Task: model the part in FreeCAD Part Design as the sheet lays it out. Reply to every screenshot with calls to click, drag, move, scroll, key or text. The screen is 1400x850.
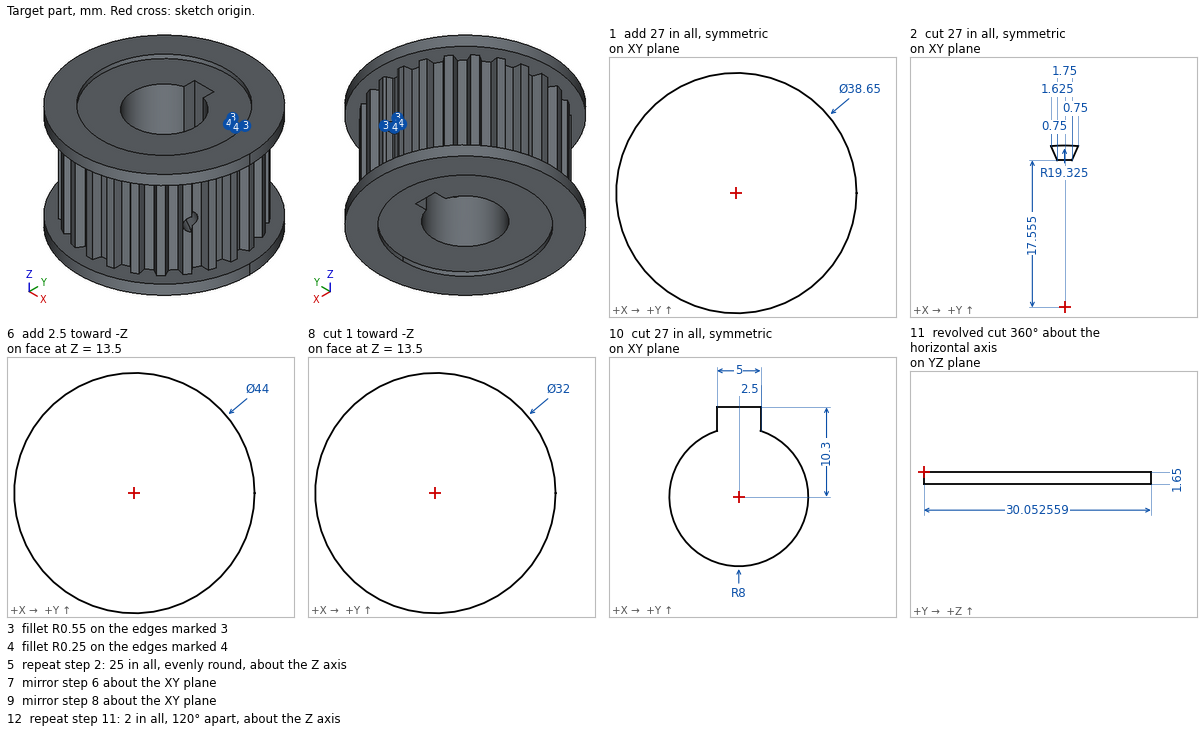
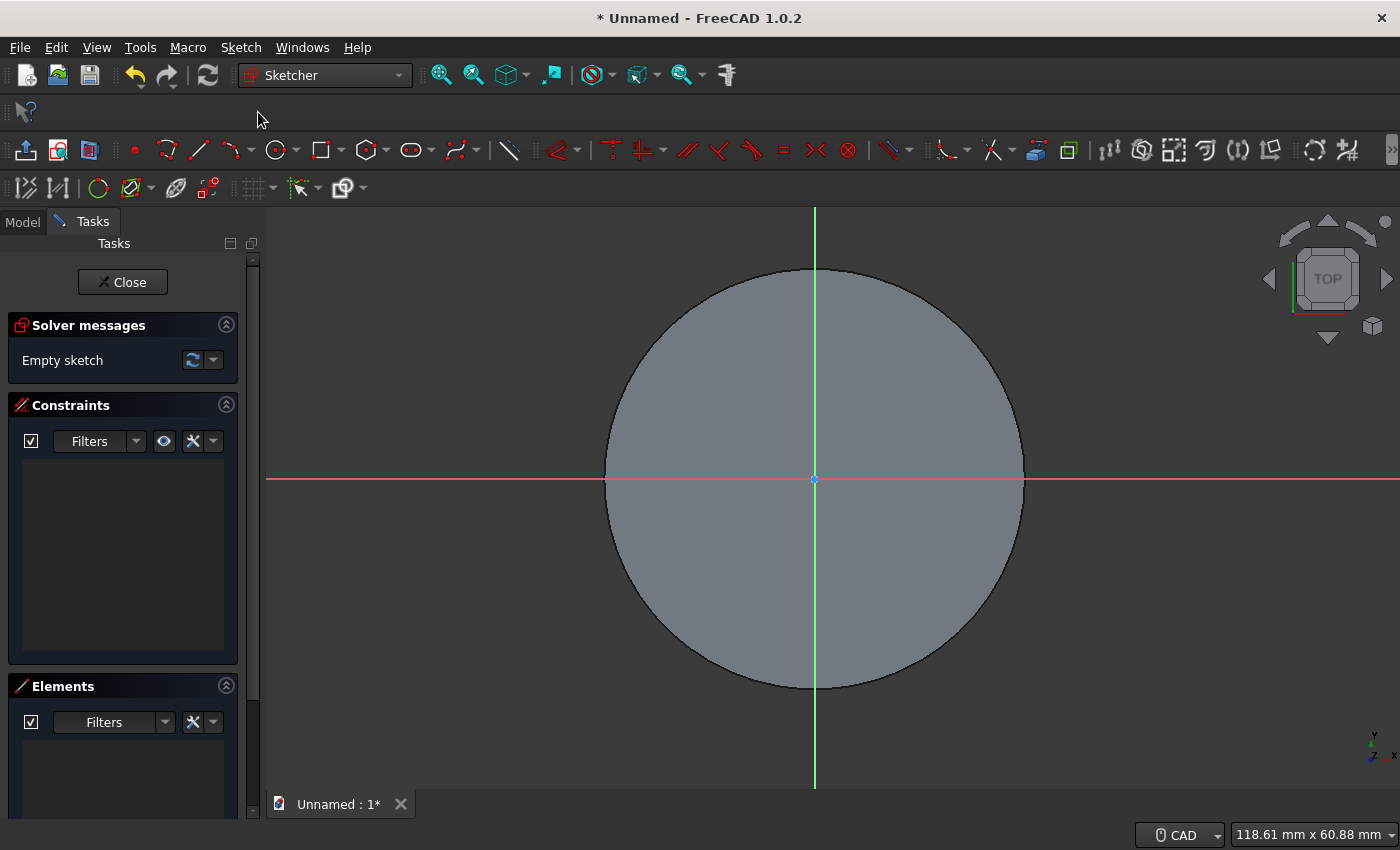
click(276, 150)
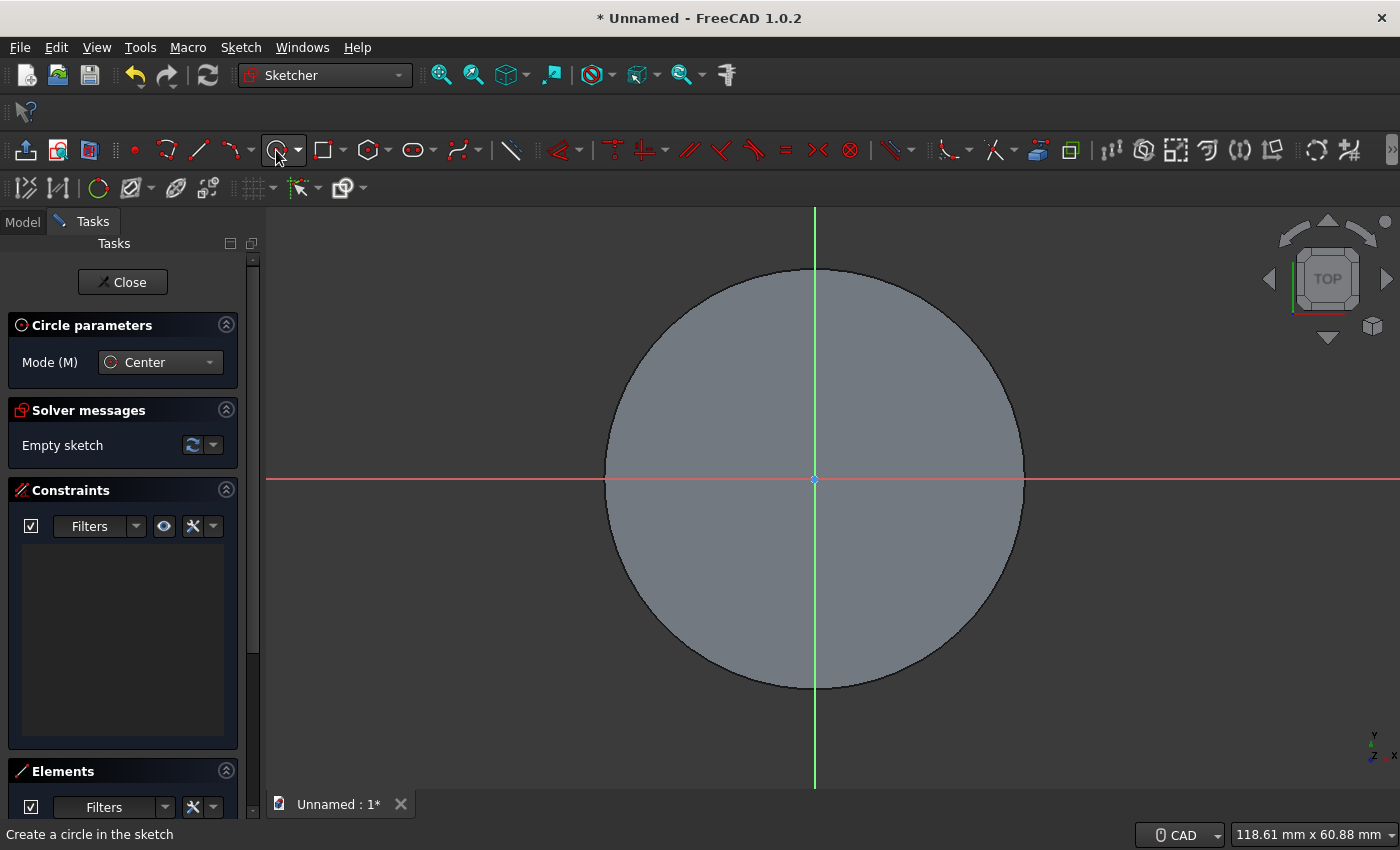
click(815, 479)
move(923, 371)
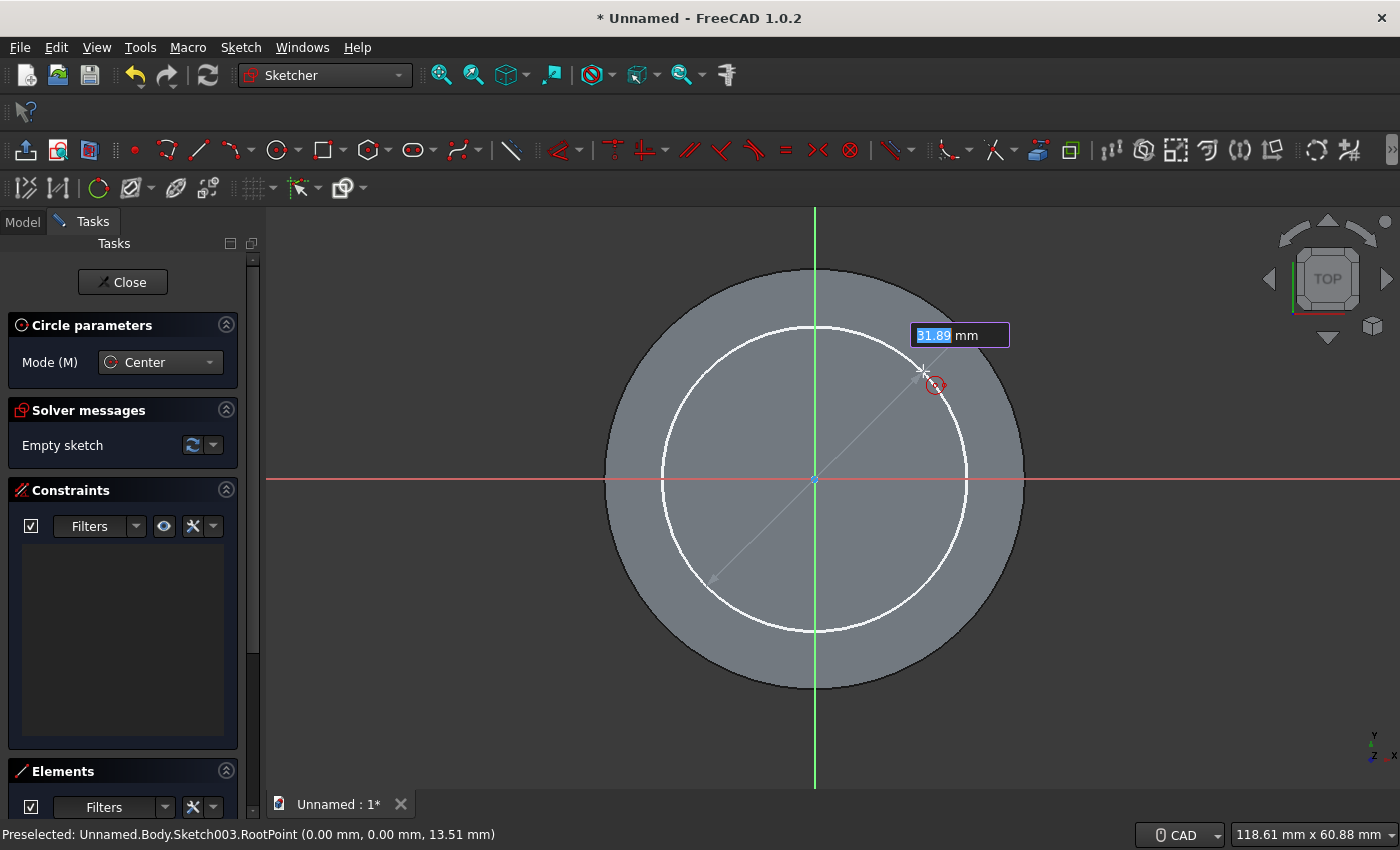
text(32)
key(Return)
key(Escape)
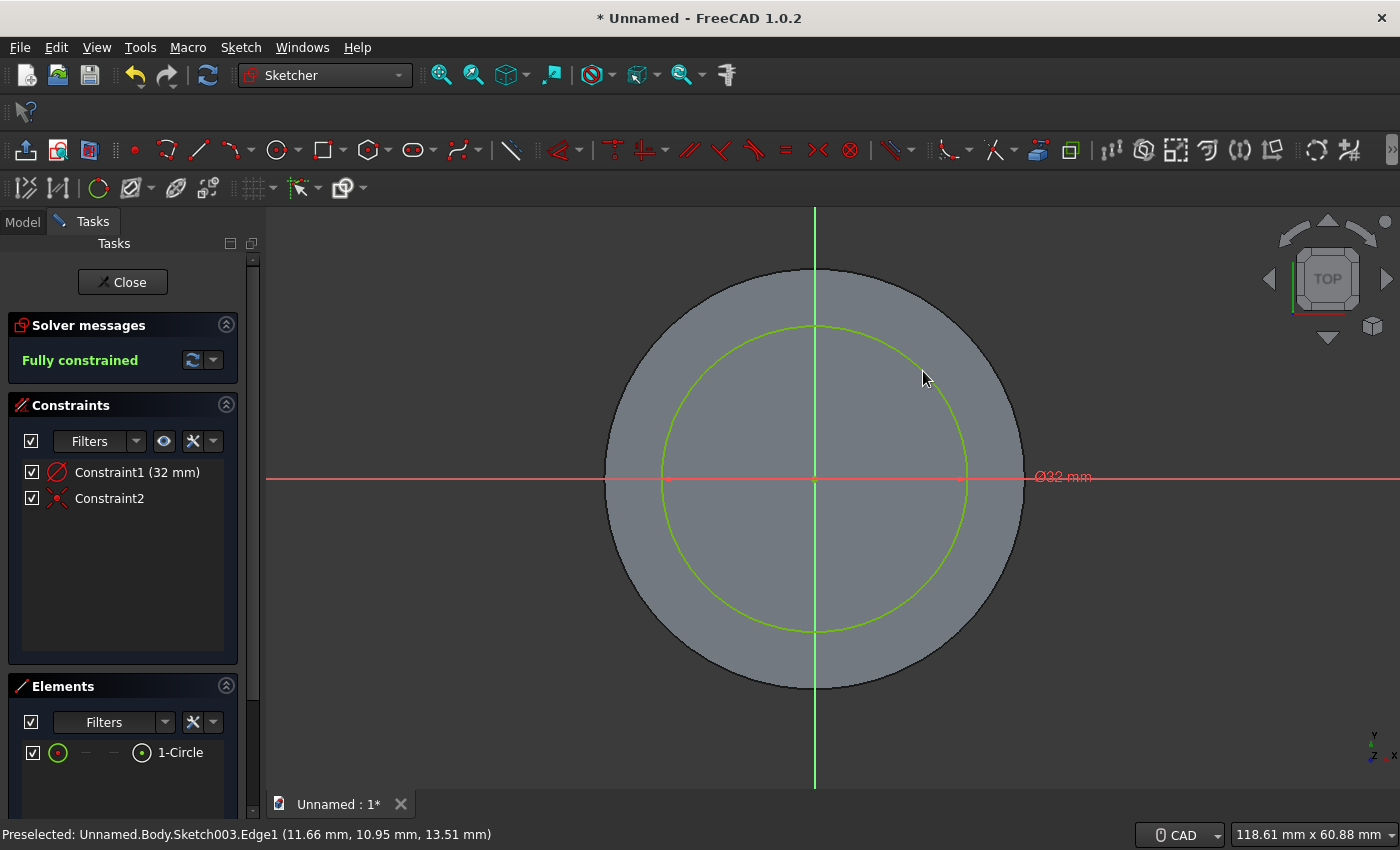
click(123, 282)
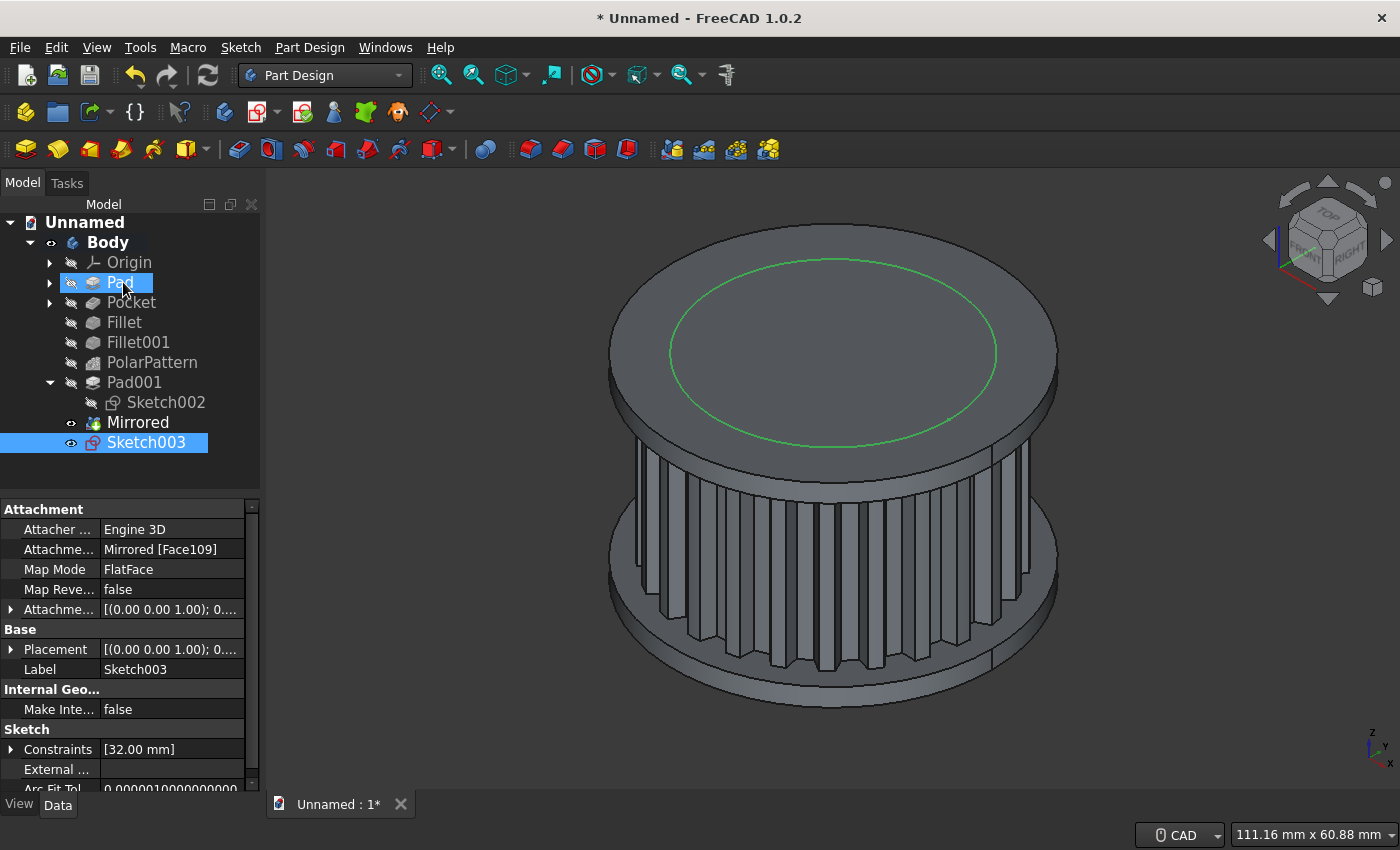
click(240, 150)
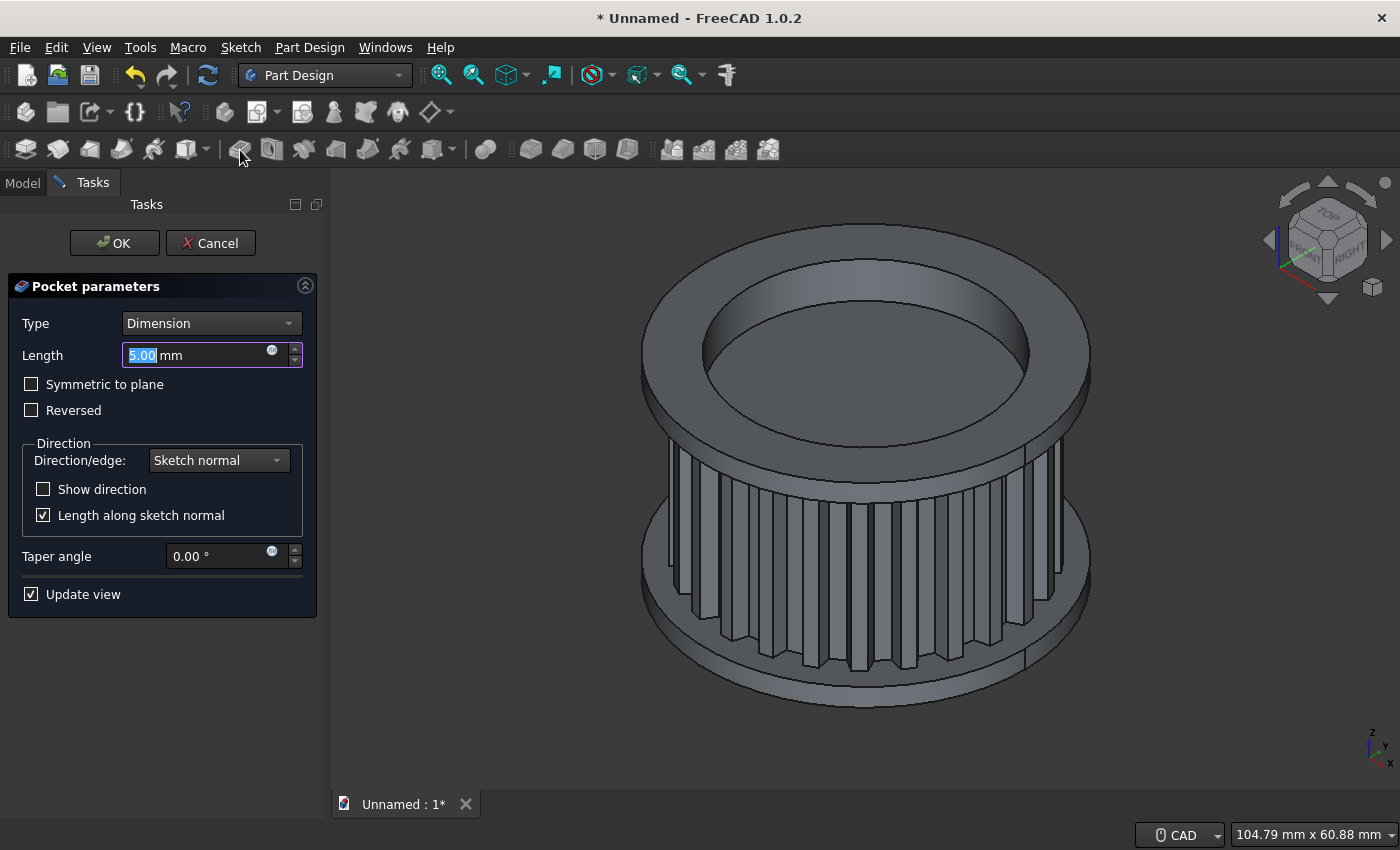
text(1)
key(Tab)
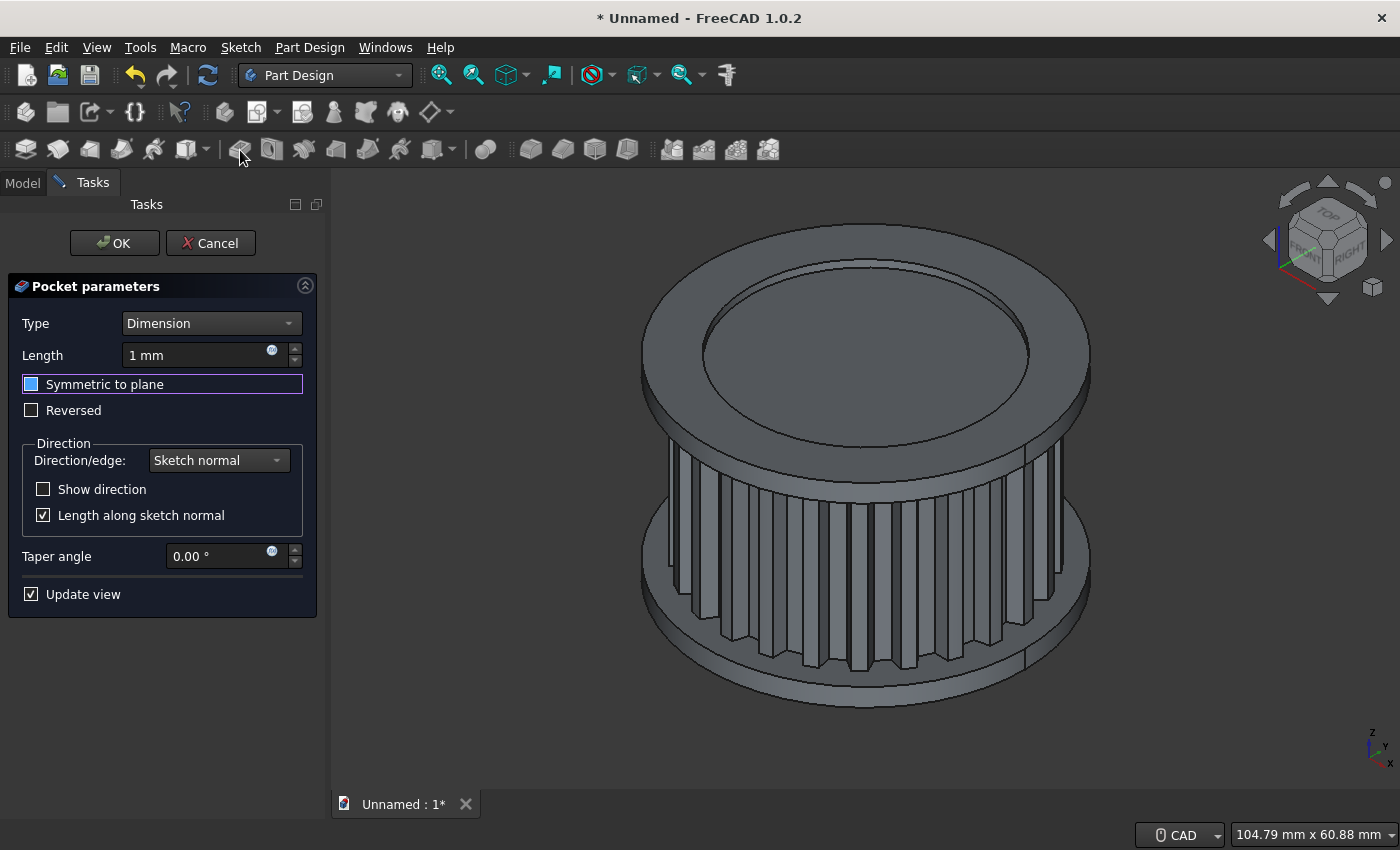
click(115, 243)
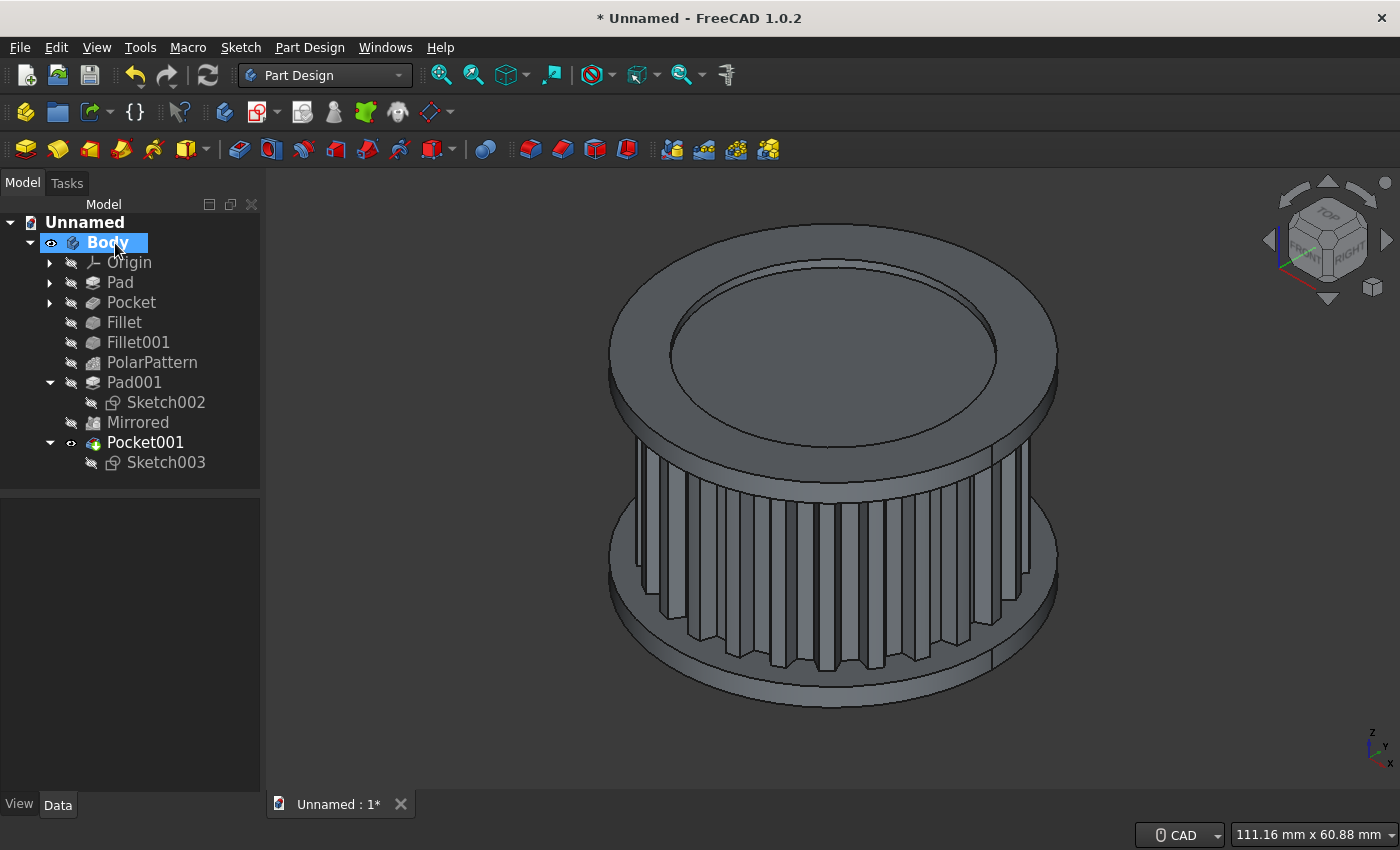
click(116, 443)